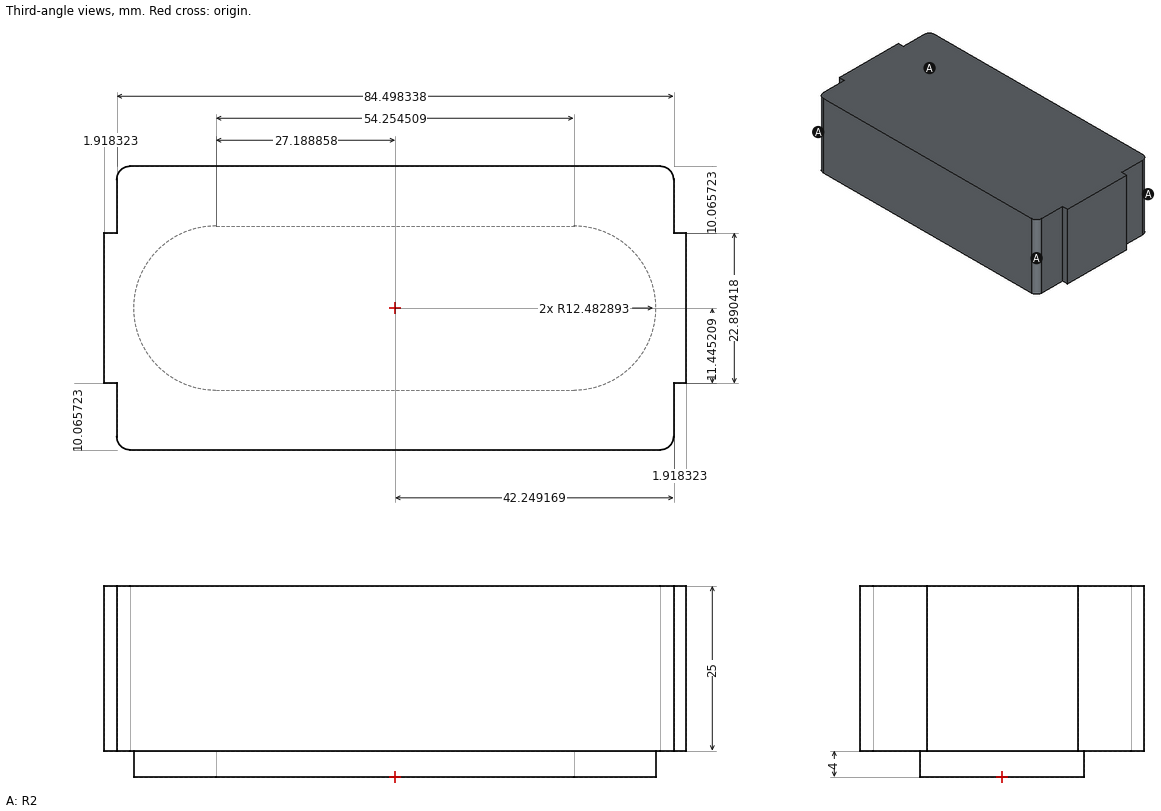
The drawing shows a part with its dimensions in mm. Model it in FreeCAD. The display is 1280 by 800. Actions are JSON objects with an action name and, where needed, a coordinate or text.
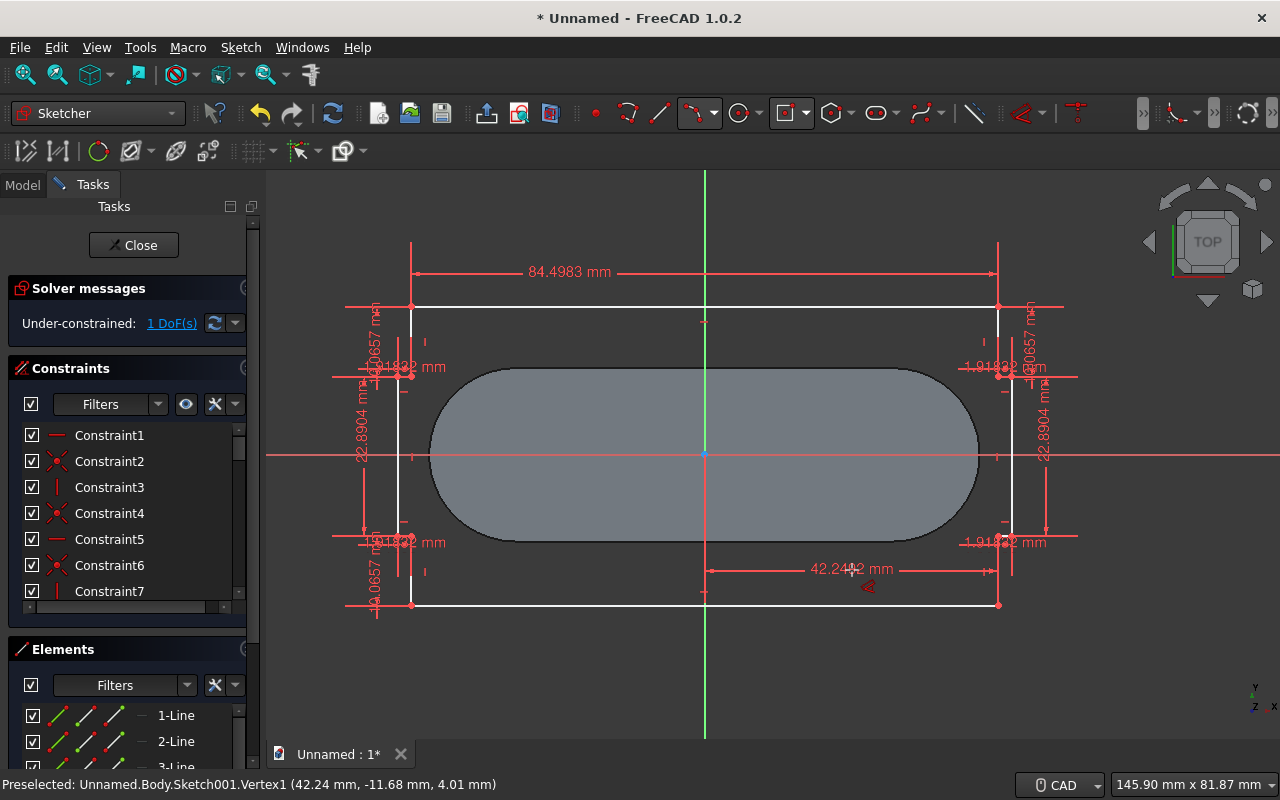
{"action": "left_click", "coordinate": [998, 536]}
{"action": "left_click", "coordinate": [1032, 495]}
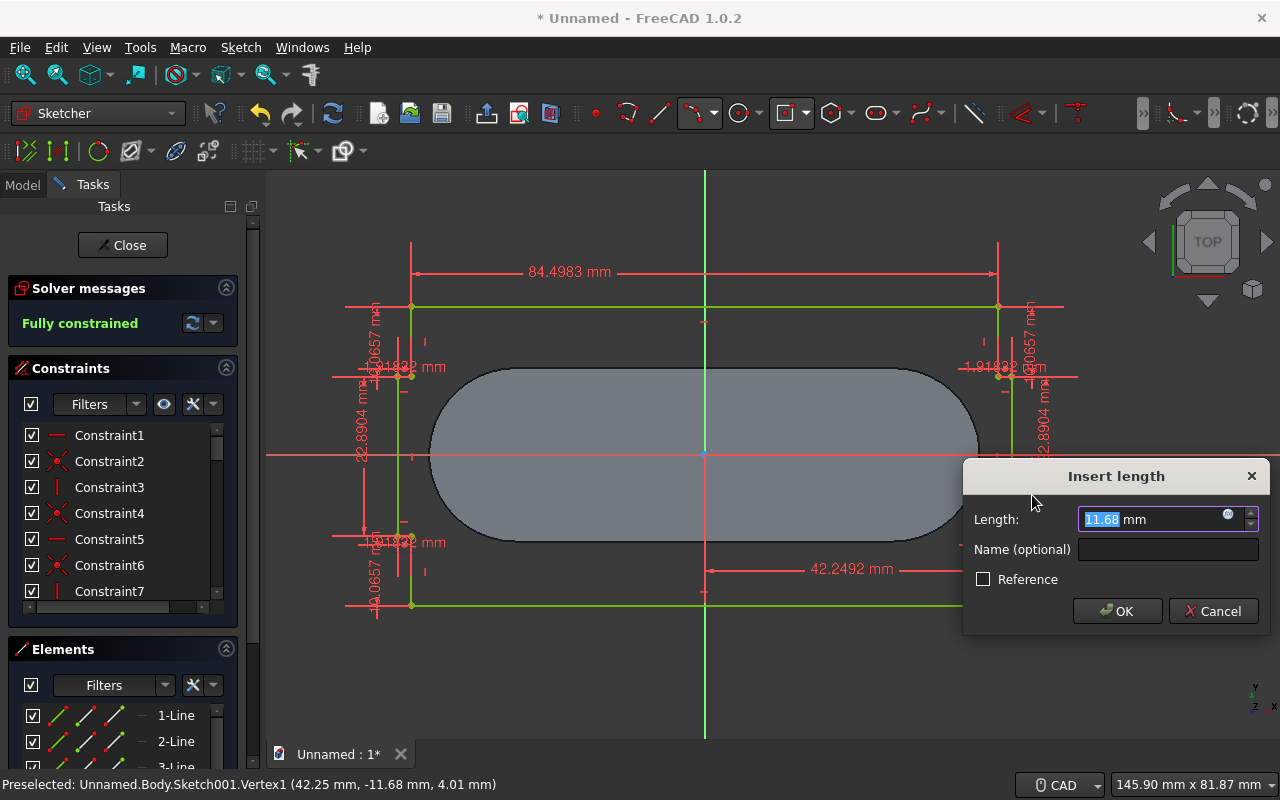
{"action": "type", "text": "11.445209"}
{"action": "key", "text": "Return"}
{"action": "key", "text": "Escape"}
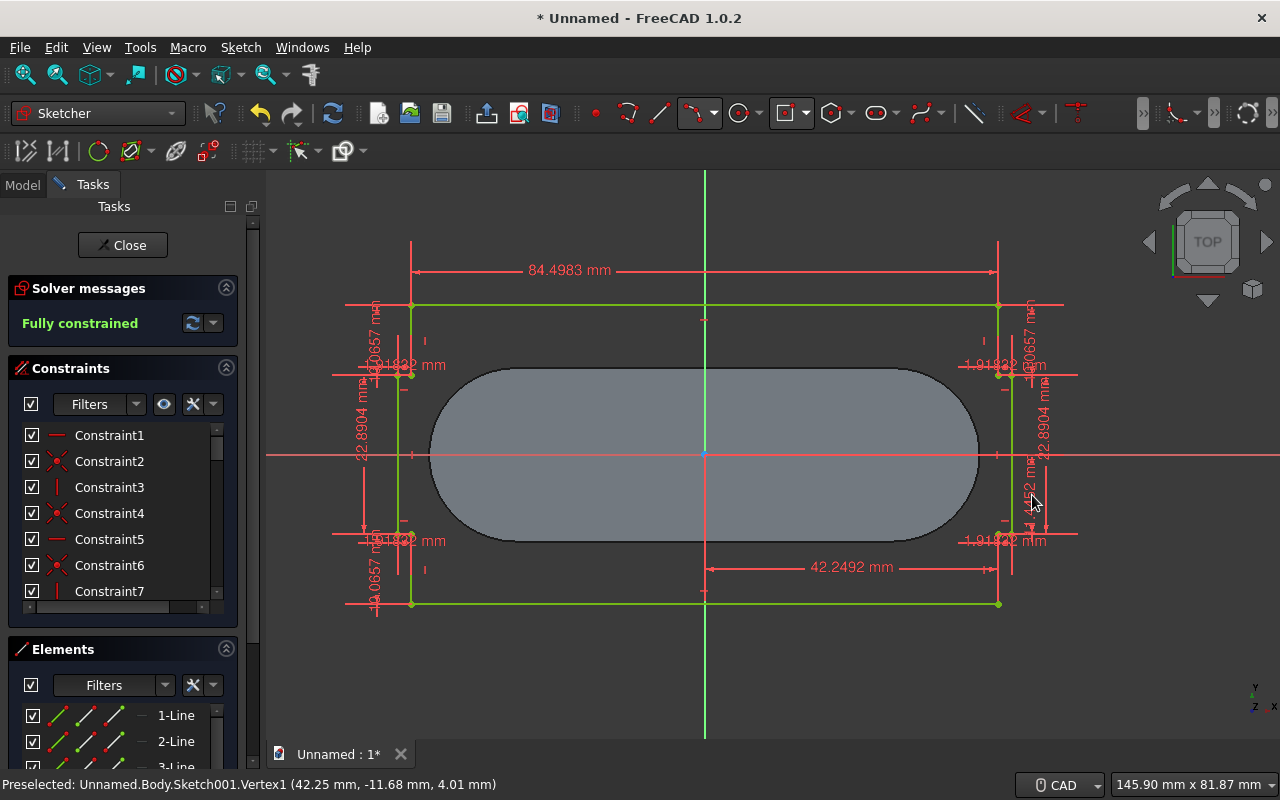
{"action": "left_click", "coordinate": [123, 245]}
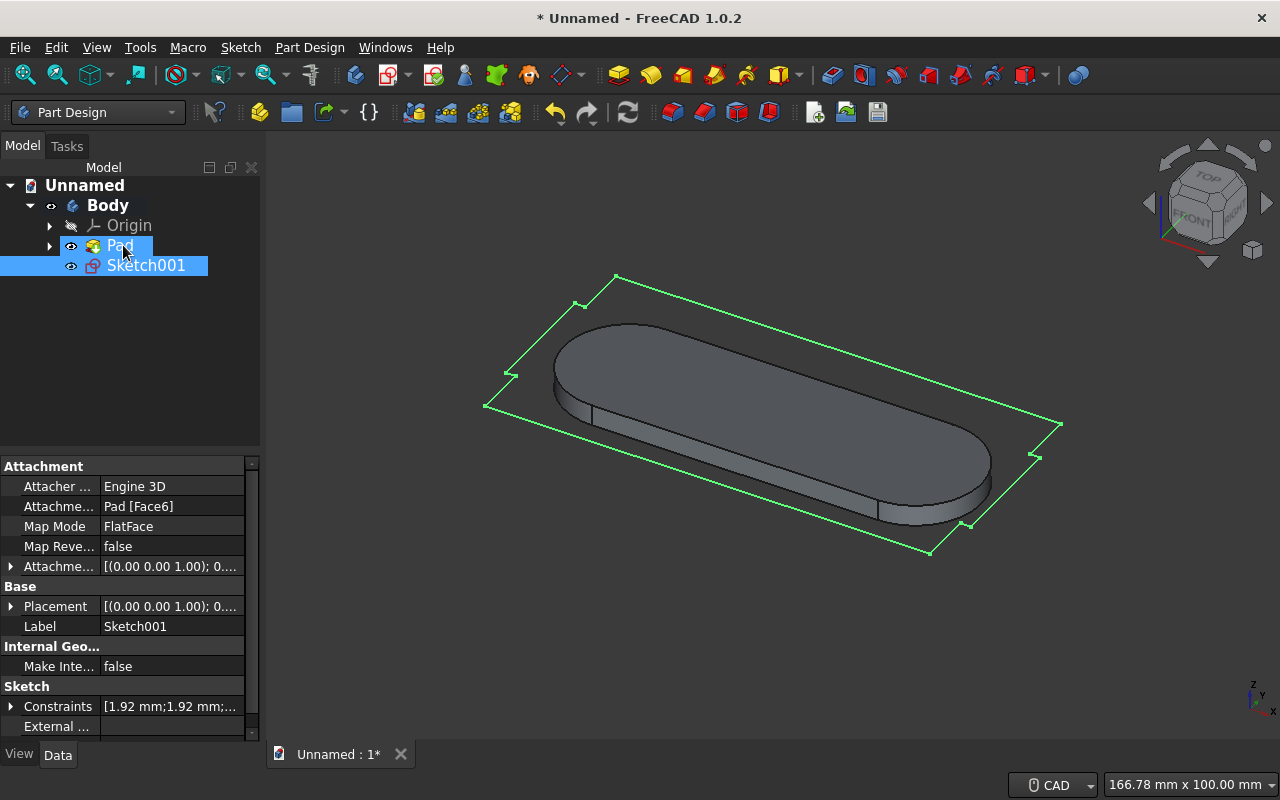
{"action": "left_click", "coordinate": [620, 76]}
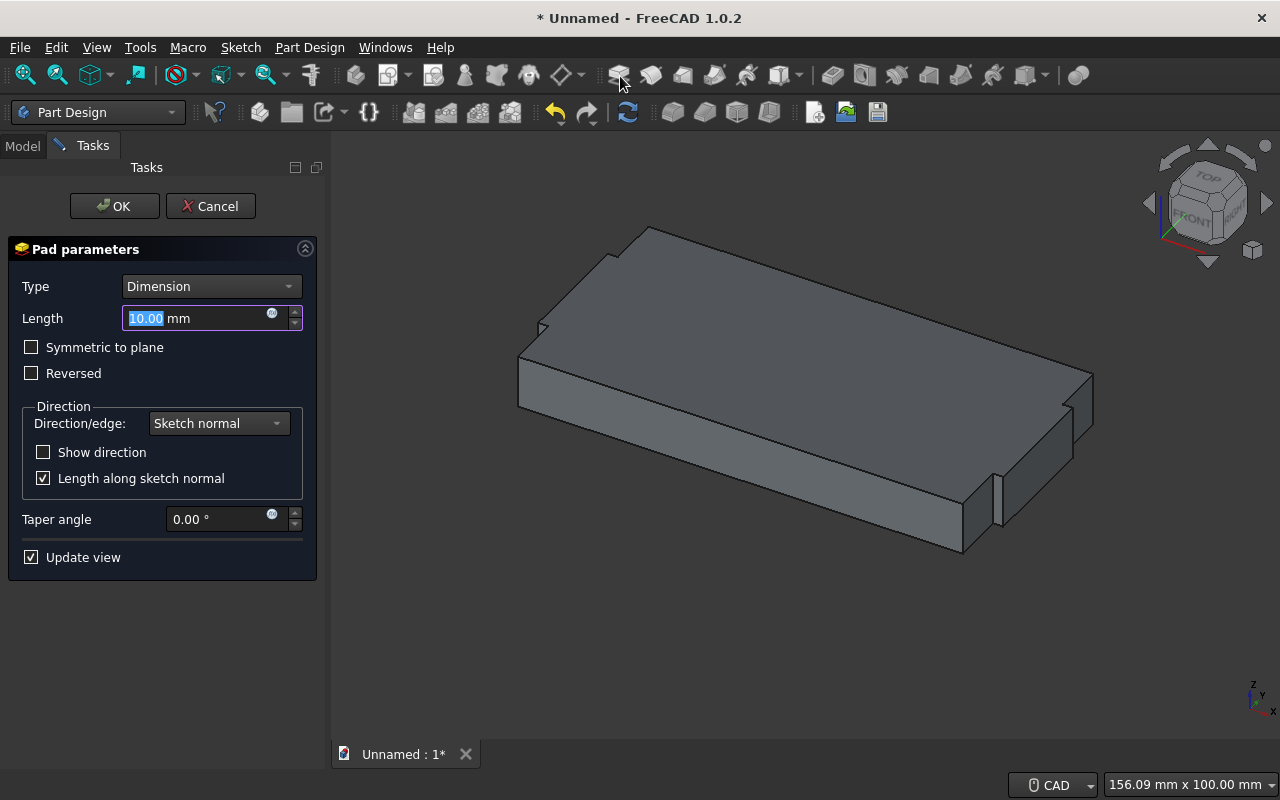
{"action": "type", "text": "25"}
{"action": "key", "text": "Tab"}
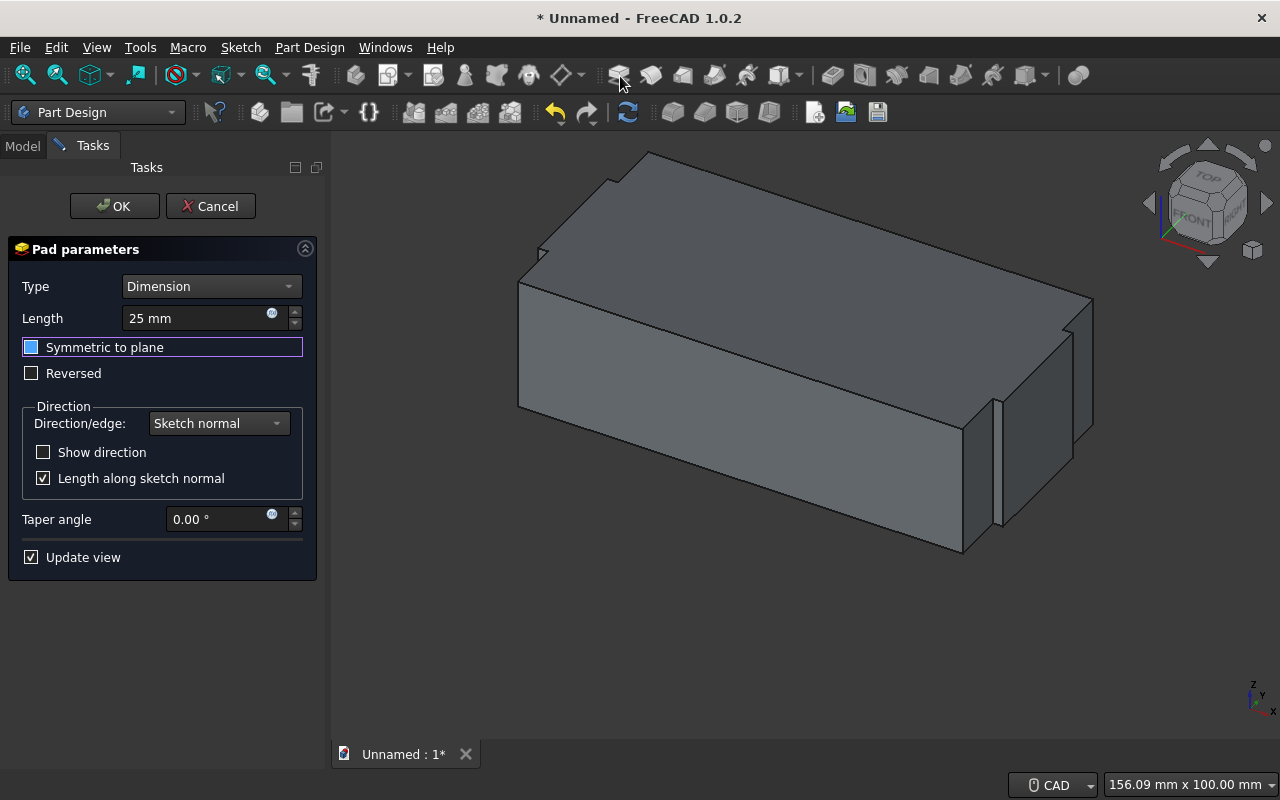
{"action": "left_click", "coordinate": [115, 206]}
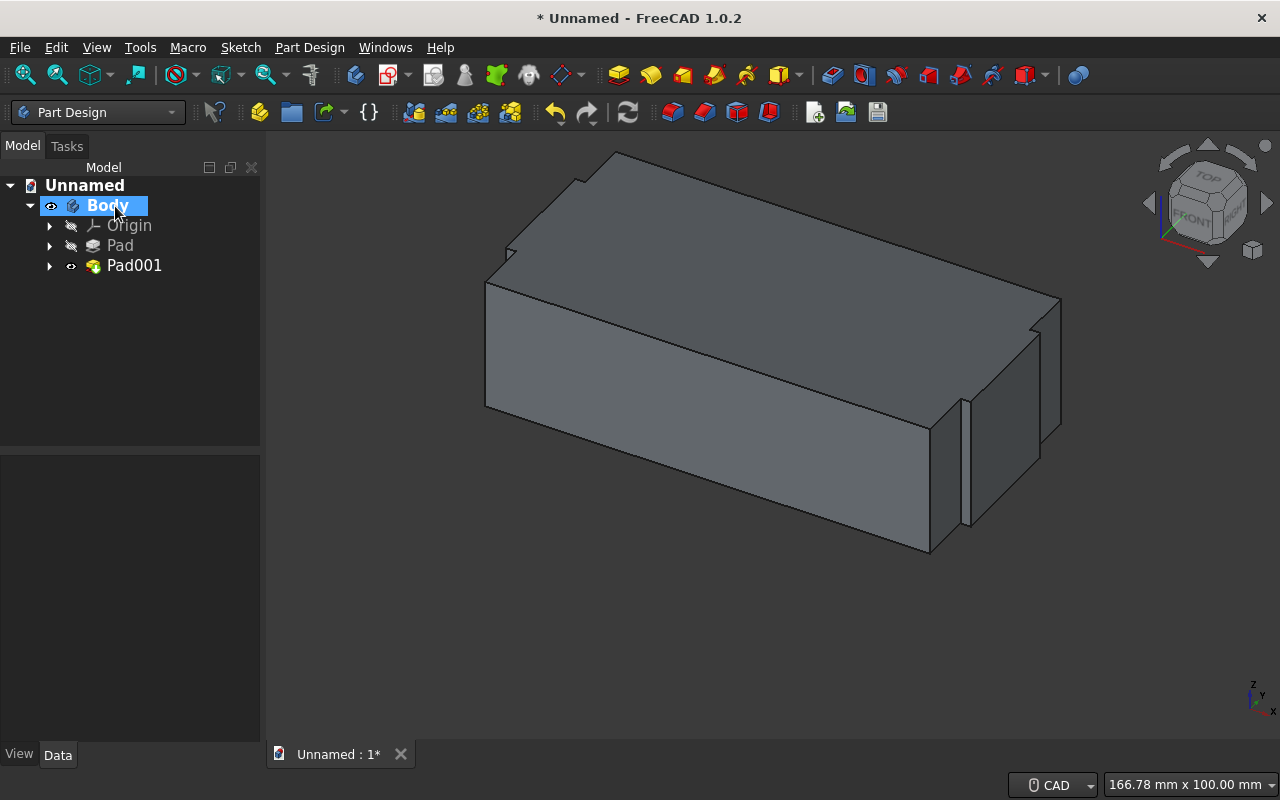
{"action": "left_click", "coordinate": [930, 490]}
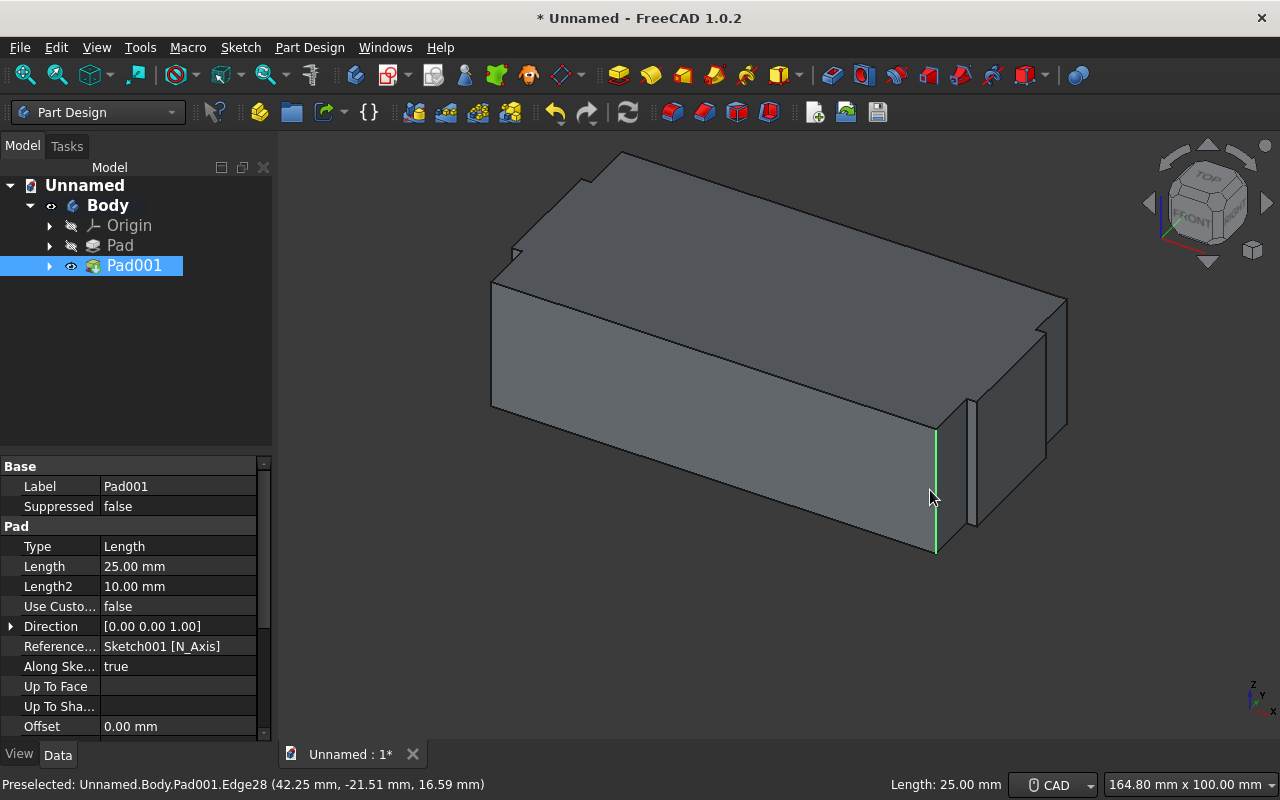
{"action": "key", "text": "0"}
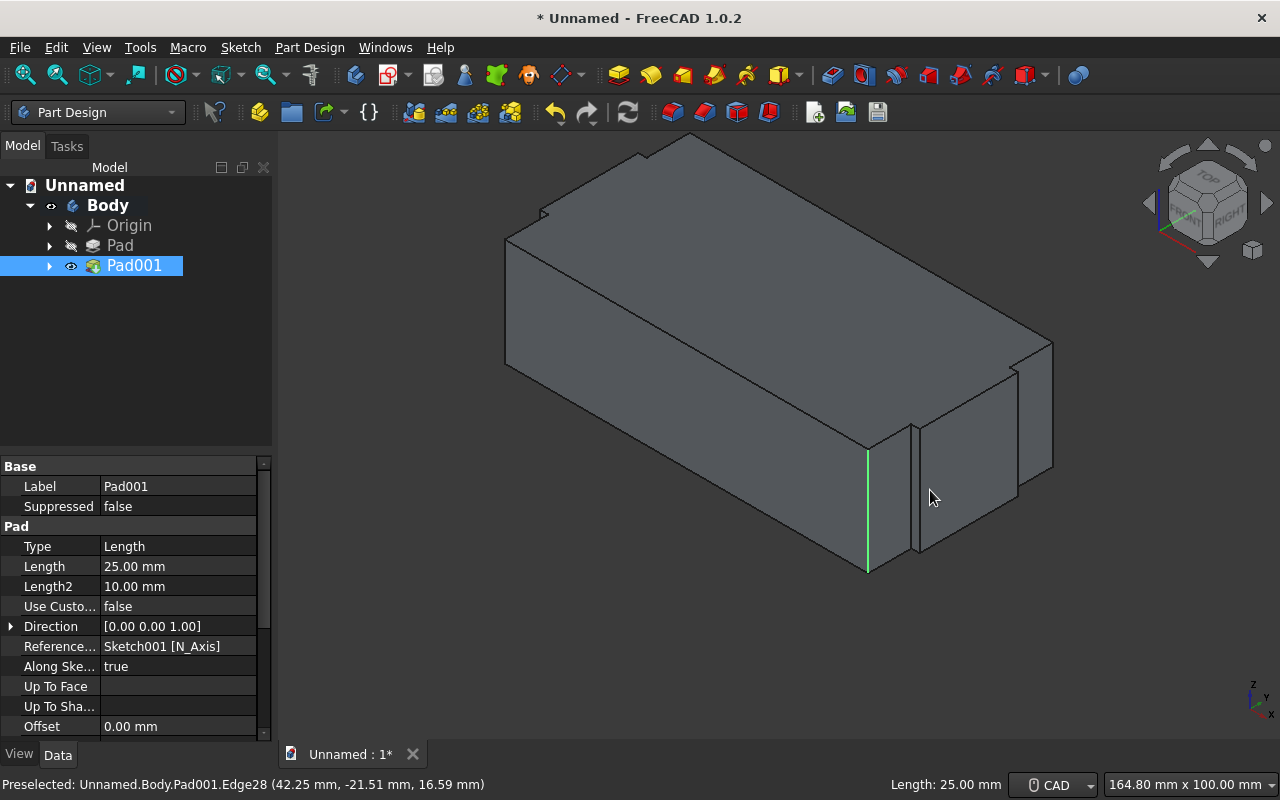
{"action": "left_click", "coordinate": [26, 76]}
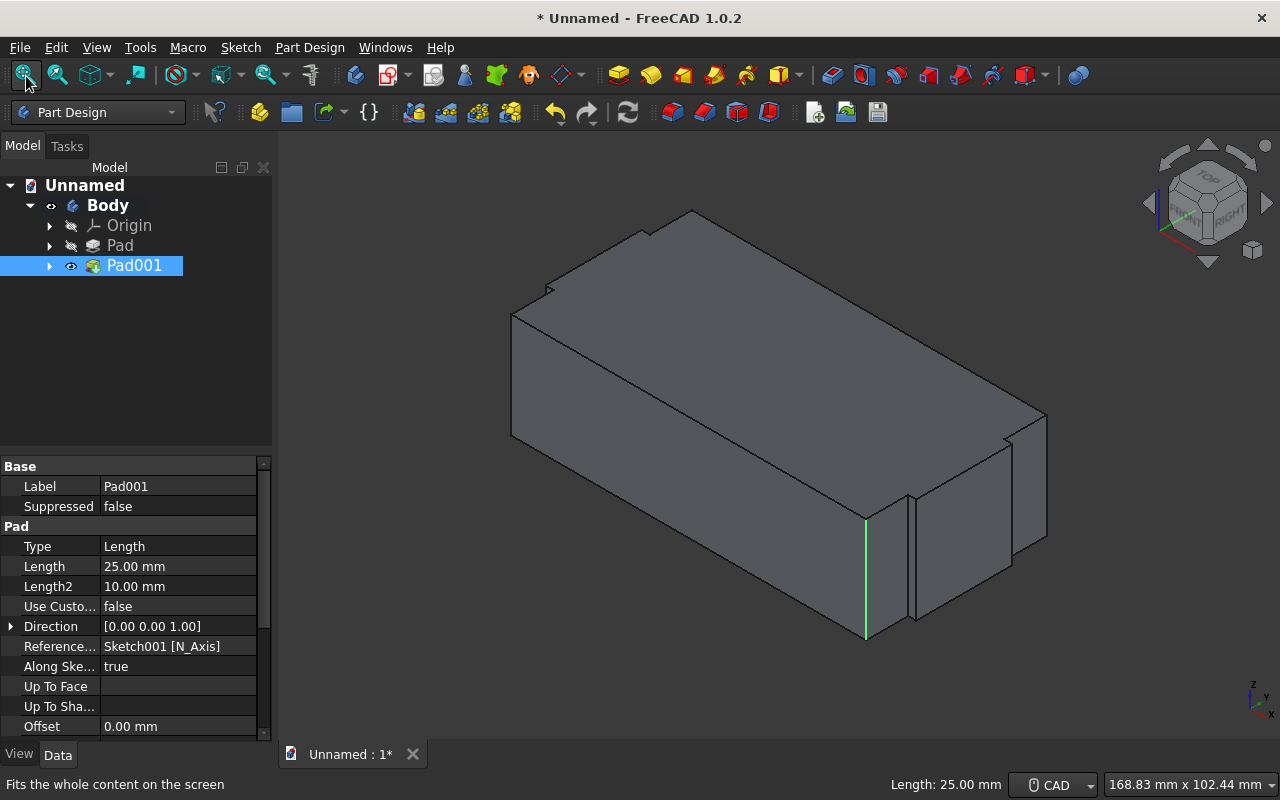
{"action": "key", "text": "2"}